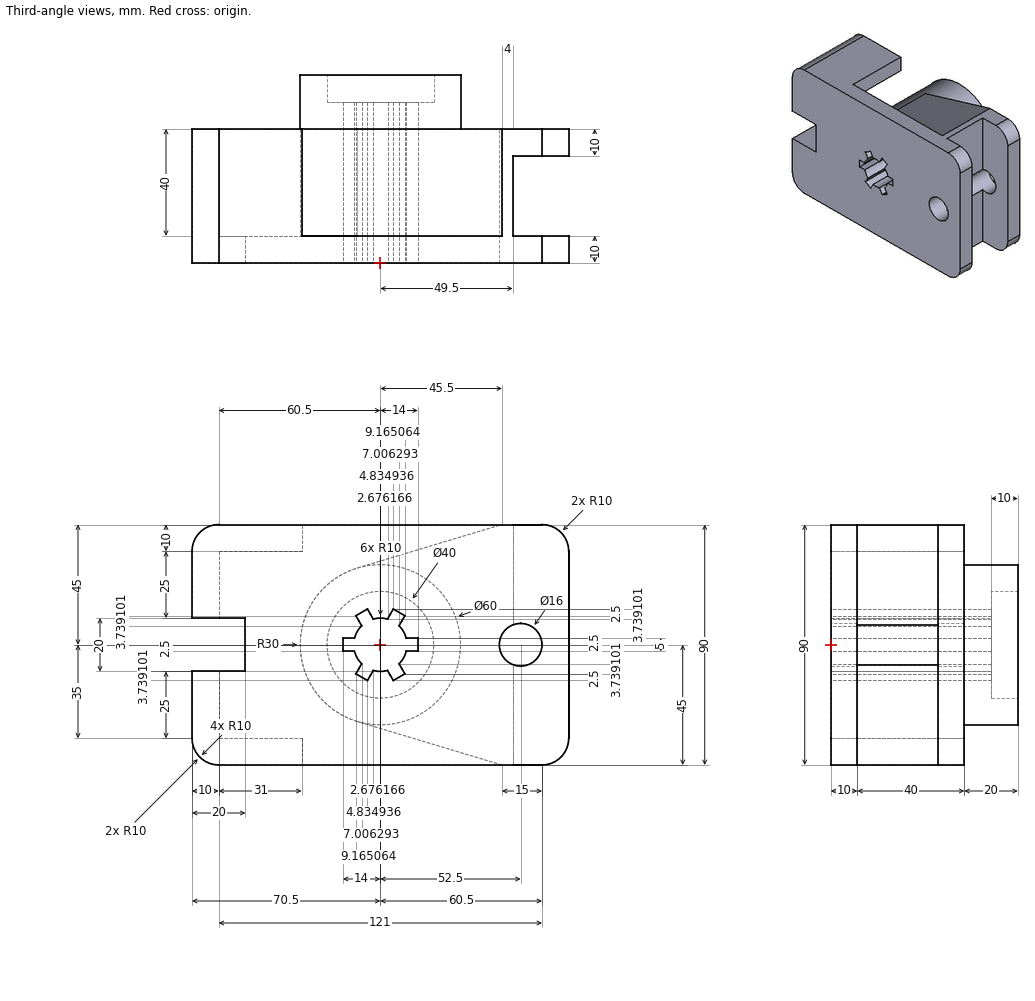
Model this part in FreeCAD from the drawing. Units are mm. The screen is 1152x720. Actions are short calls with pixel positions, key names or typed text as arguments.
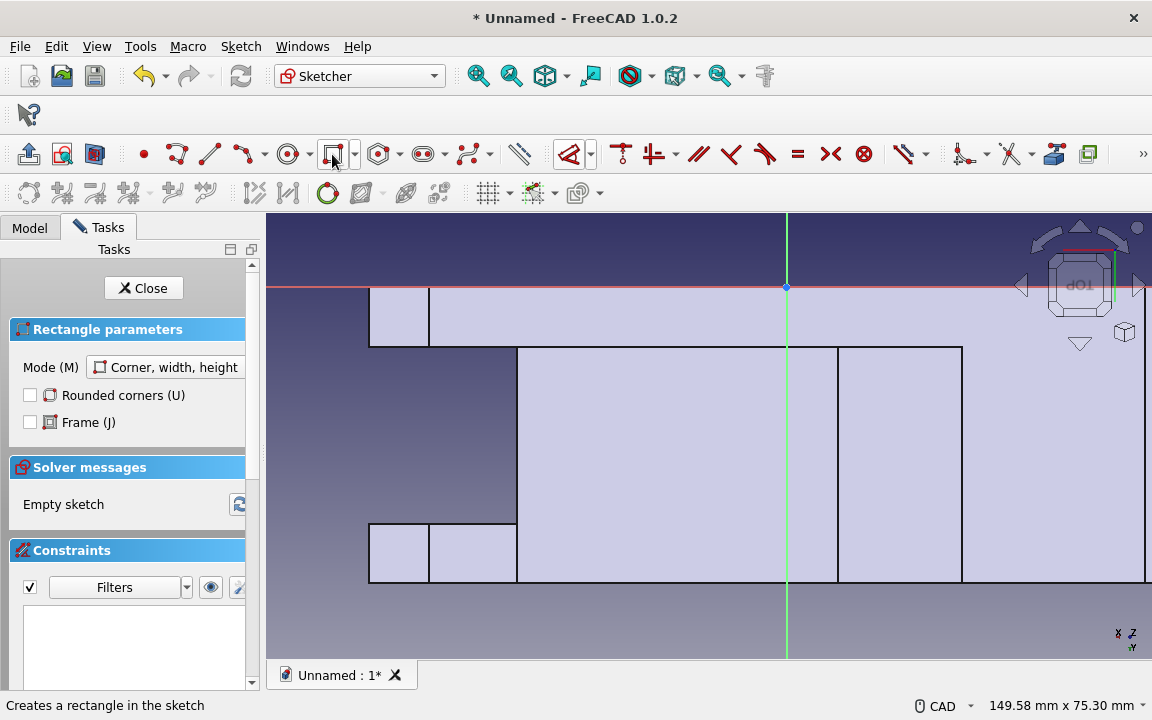
click(494, 347)
move(517, 583)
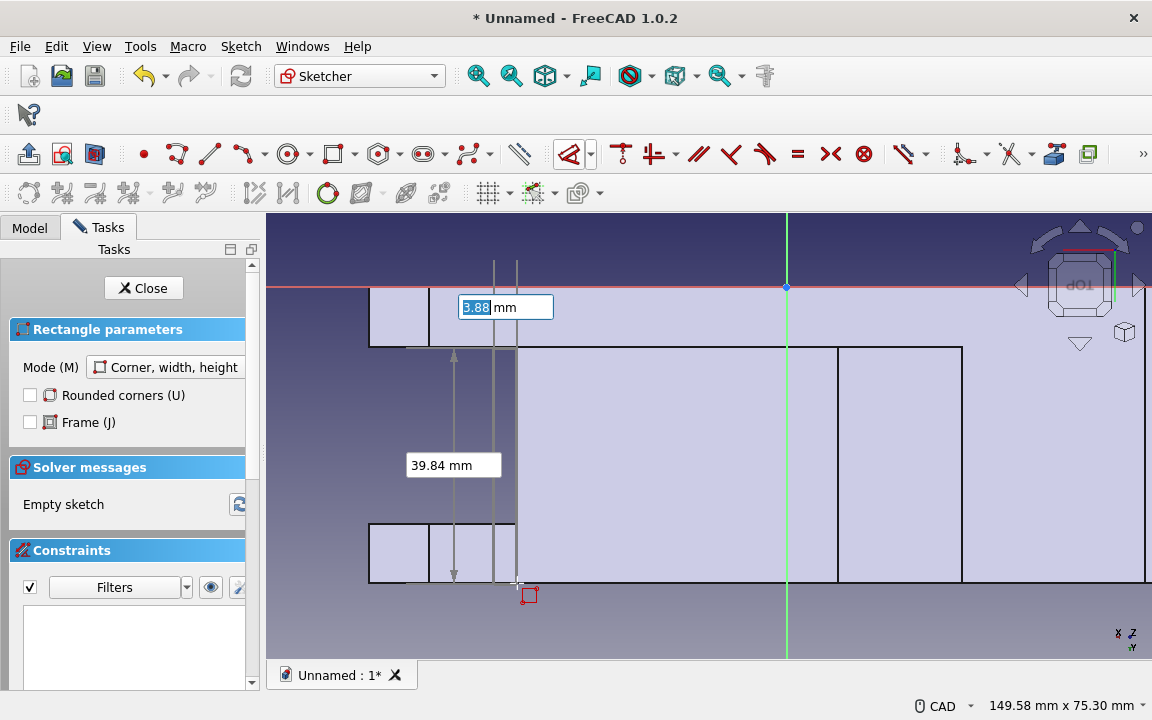
text(4)
key(Tab)
text(40)
key(Return)
key(Escape)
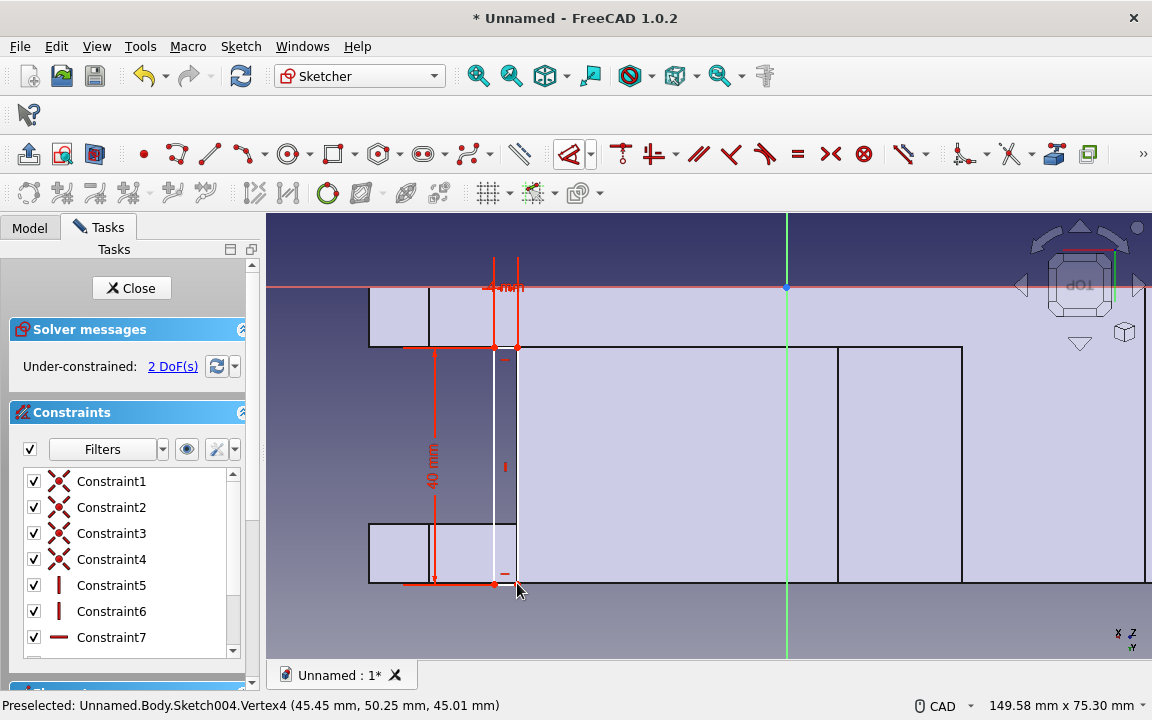
click(494, 348)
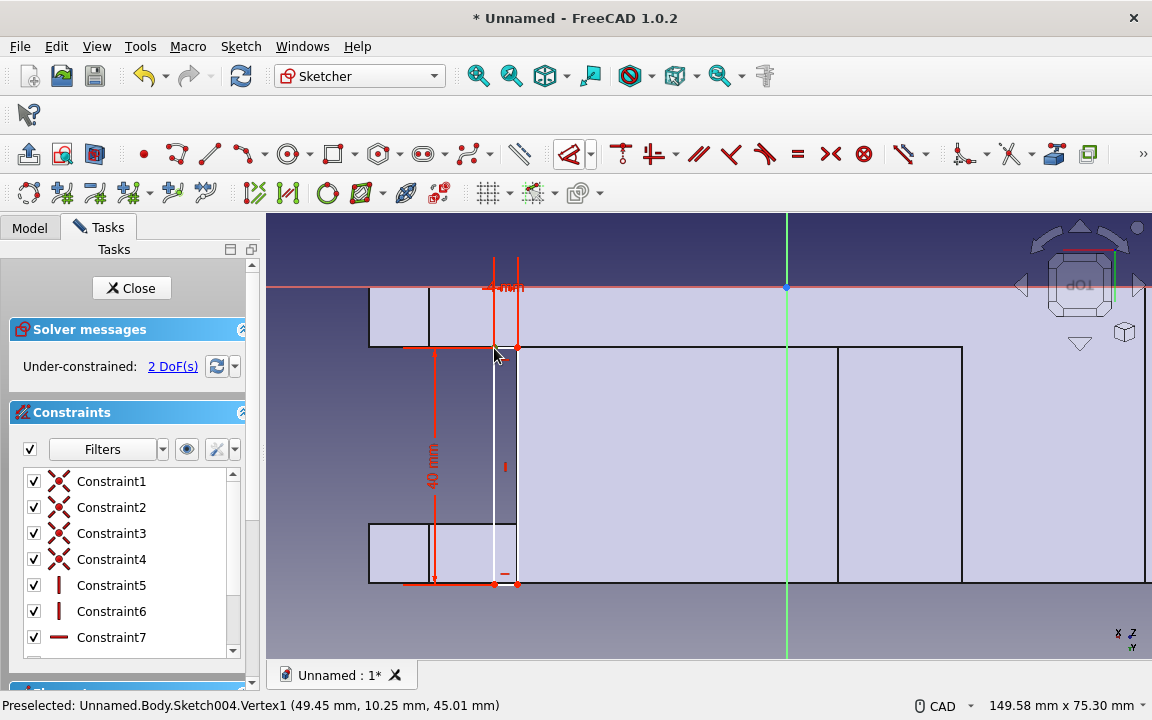
key(i)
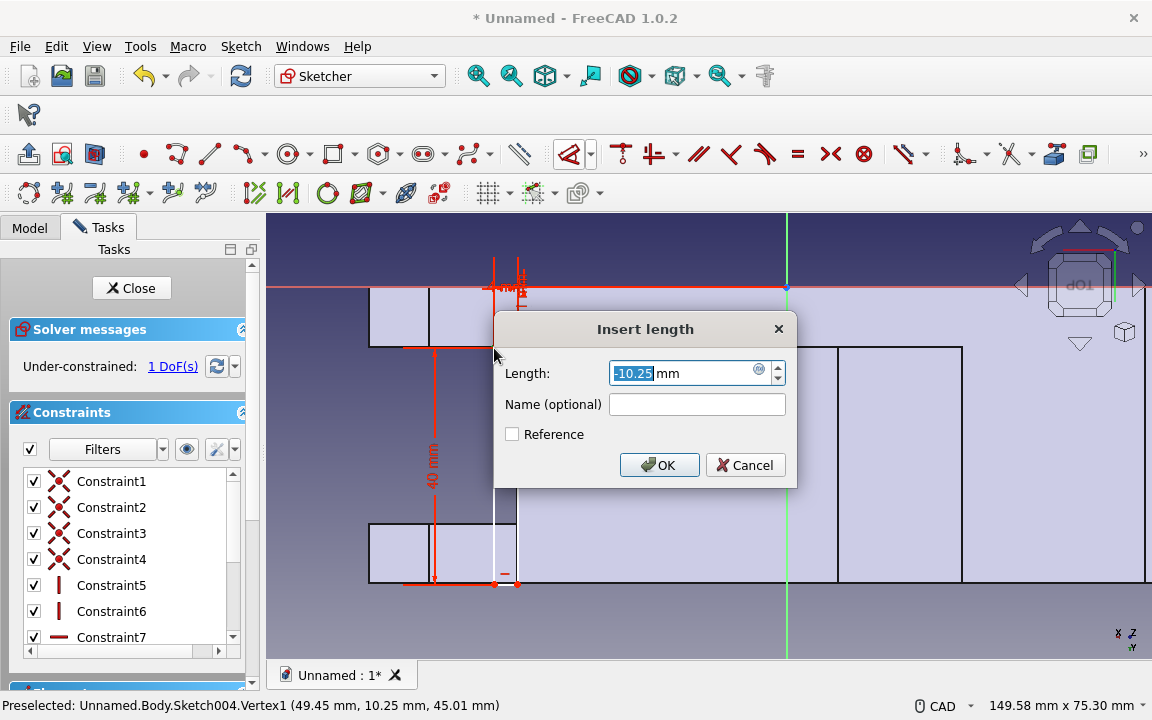
text(-10)
key(Return)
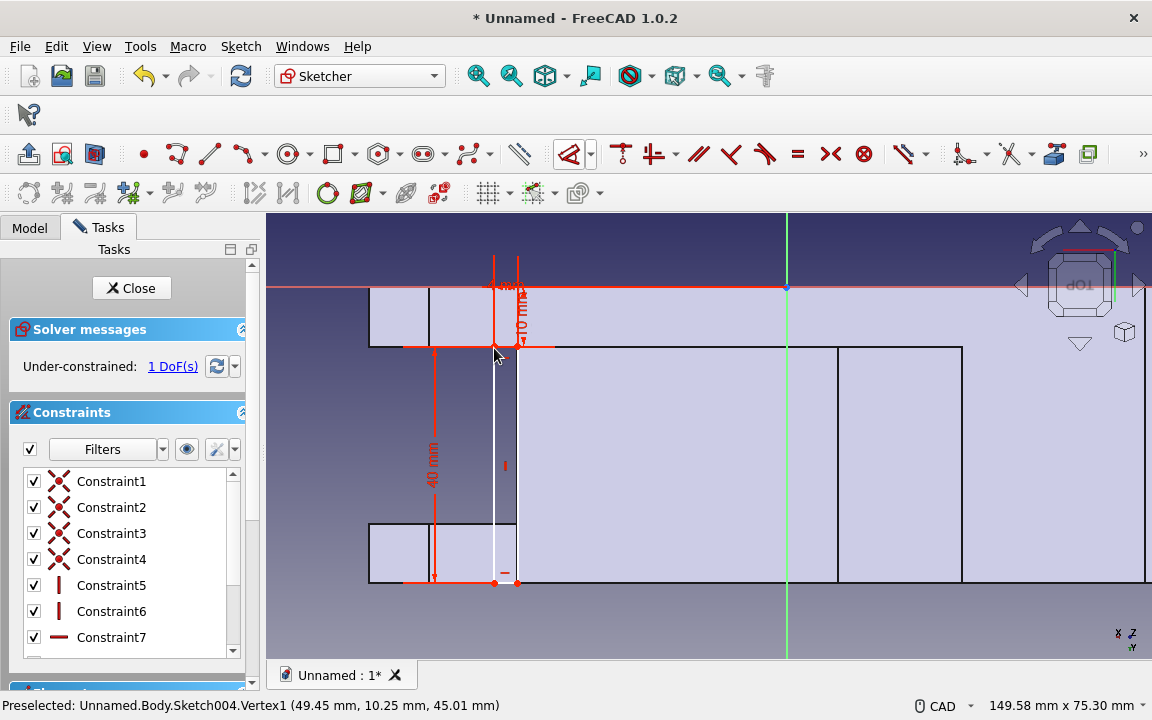
click(494, 347)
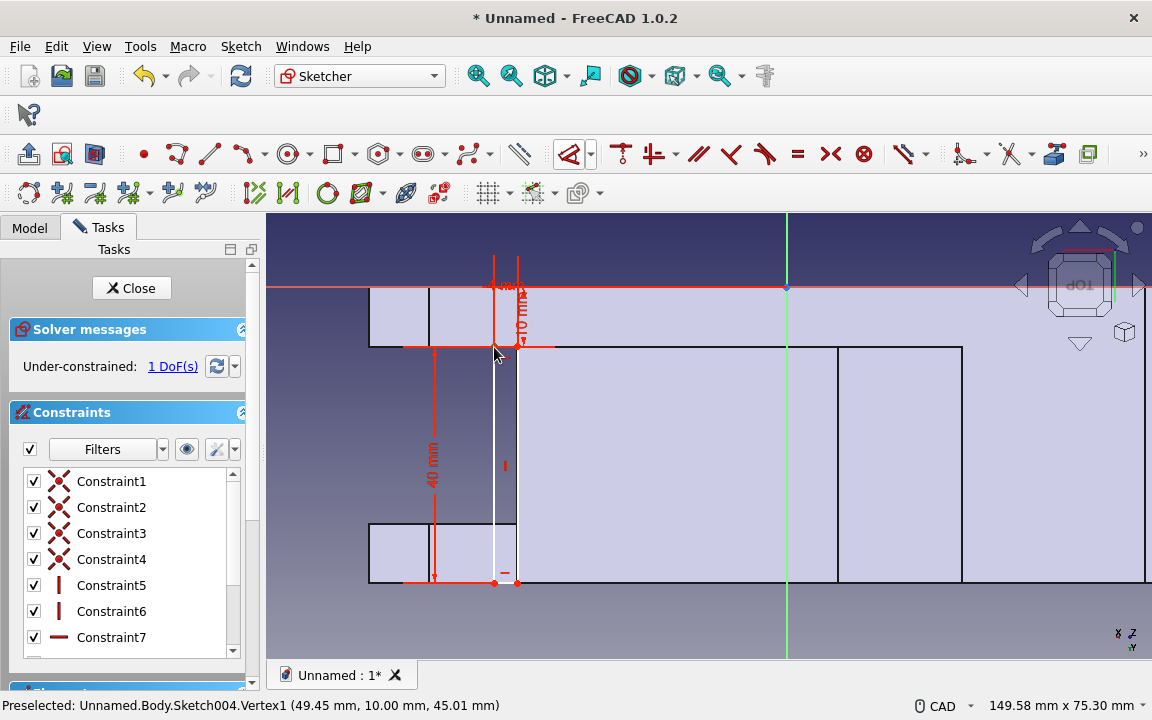
click(590, 154)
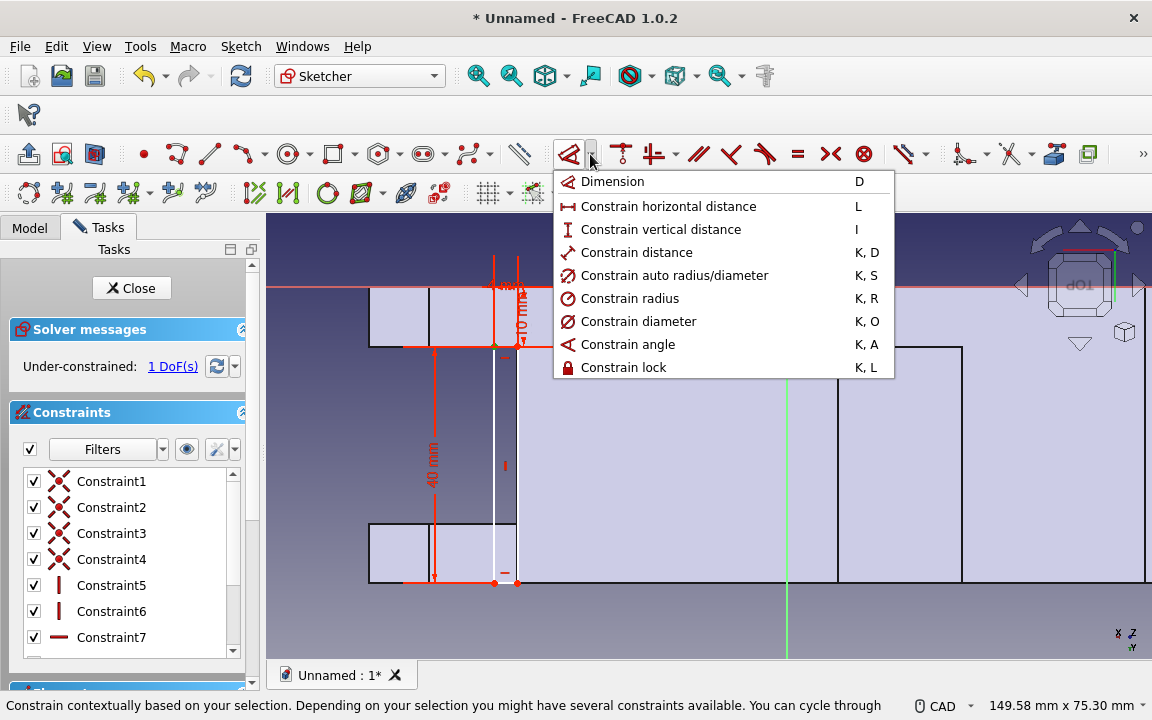
click(724, 206)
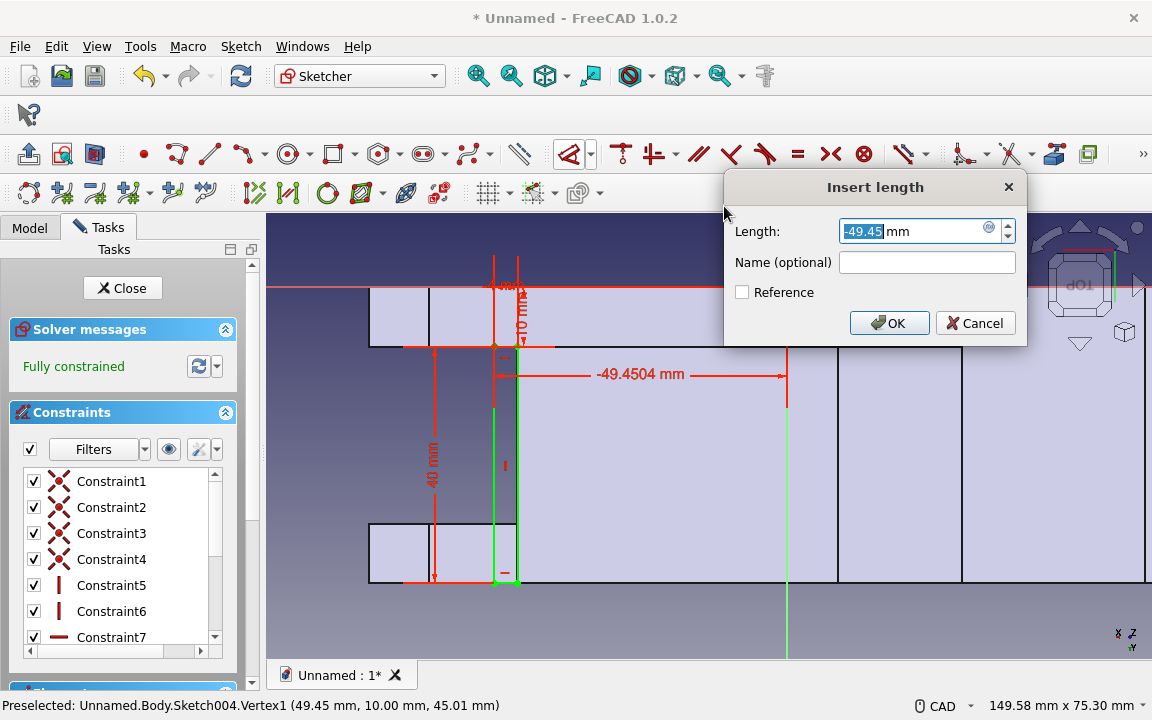
text(-49.5)
key(Return)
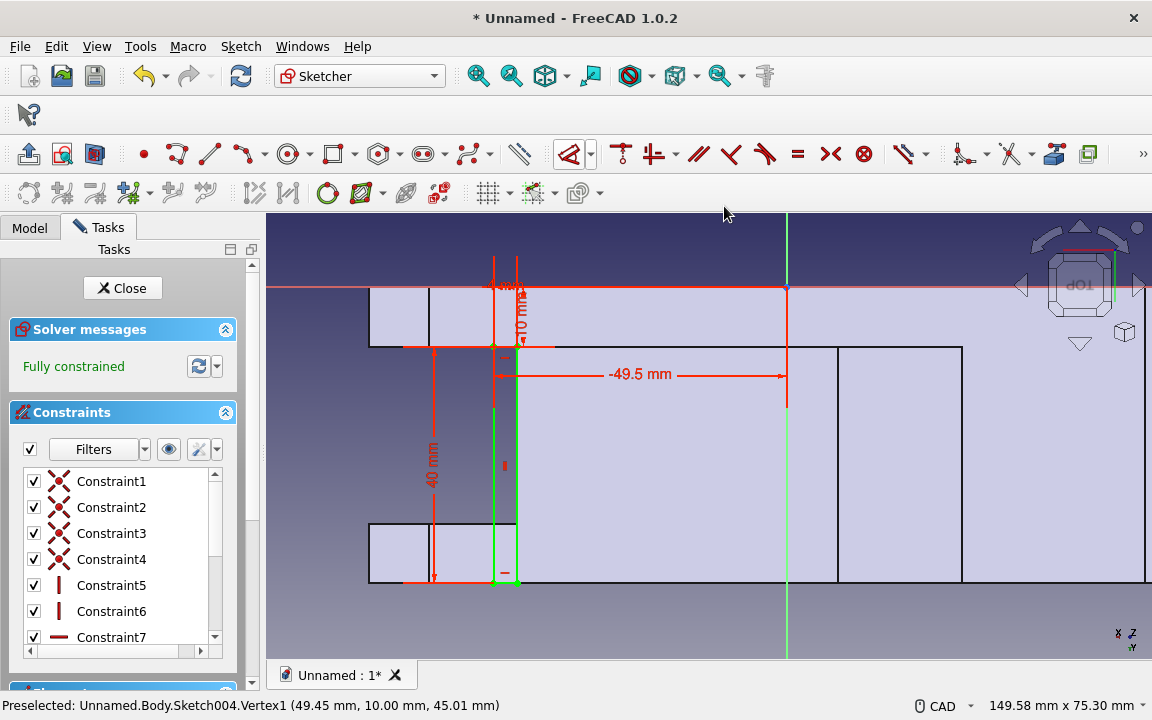
click(123, 288)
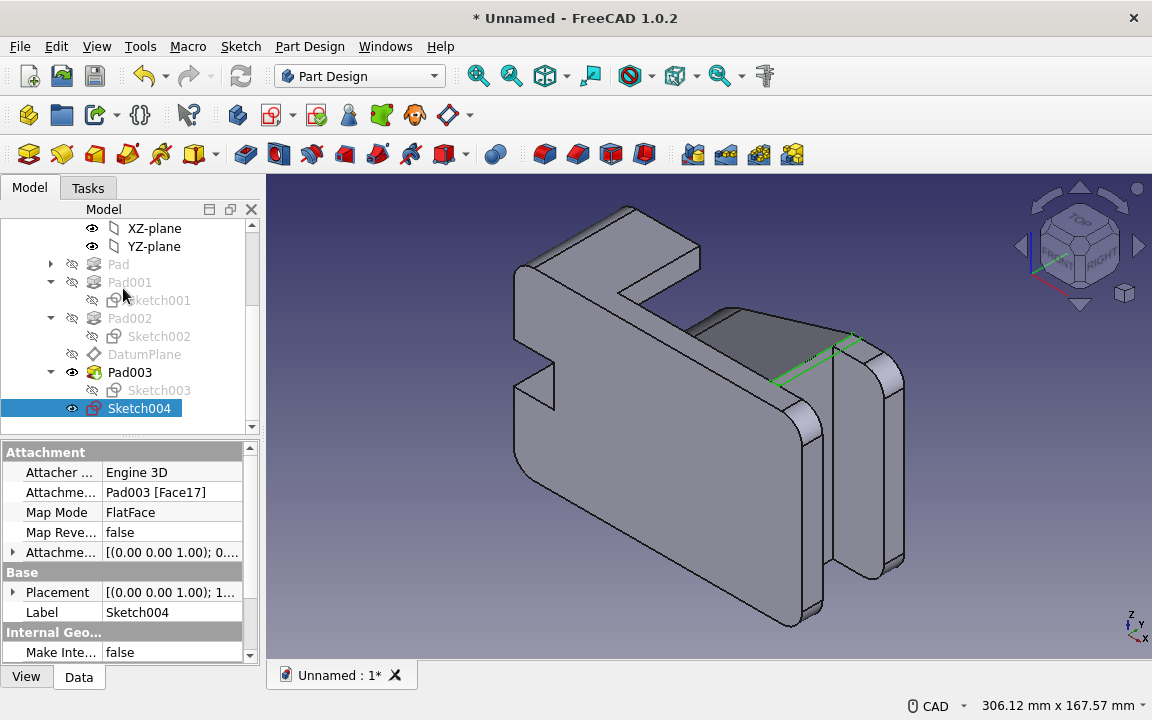
click(29, 154)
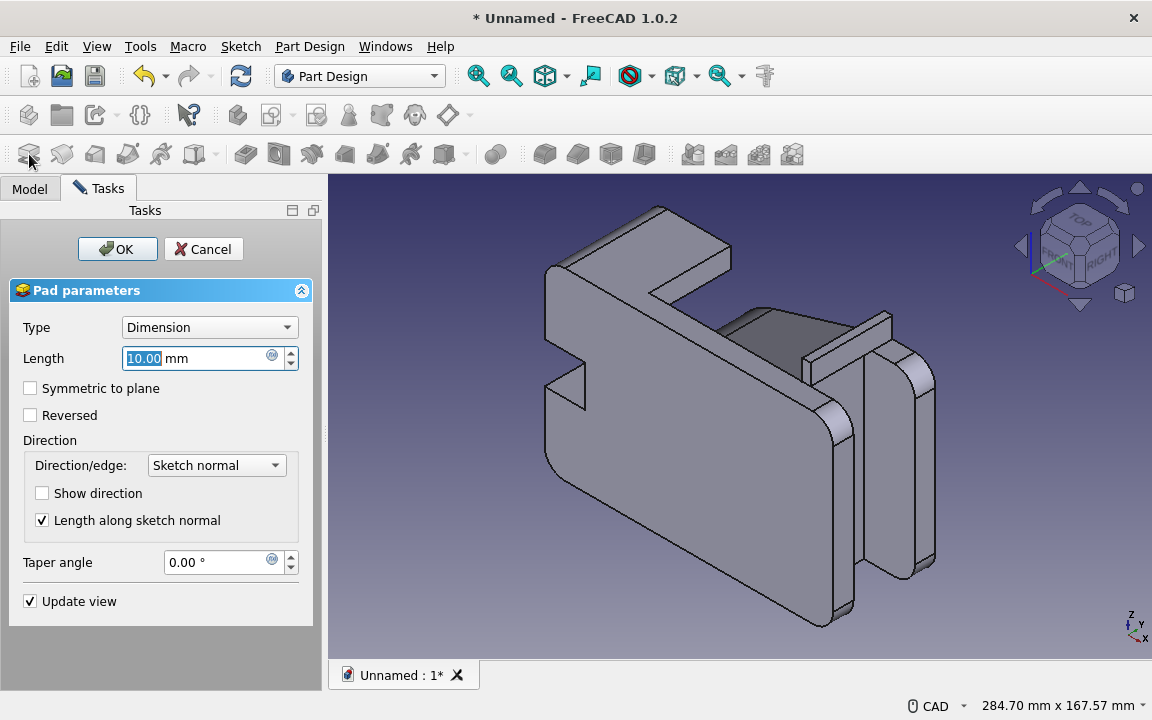
text(90)
key(Tab)